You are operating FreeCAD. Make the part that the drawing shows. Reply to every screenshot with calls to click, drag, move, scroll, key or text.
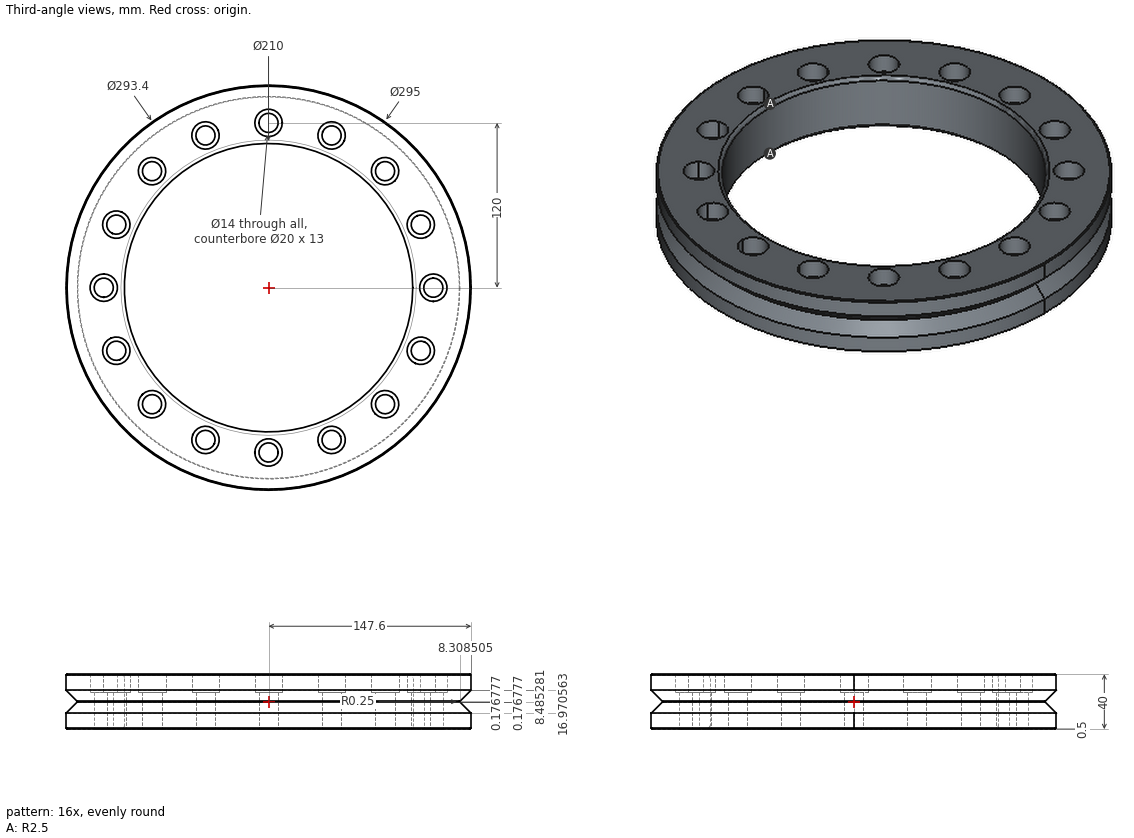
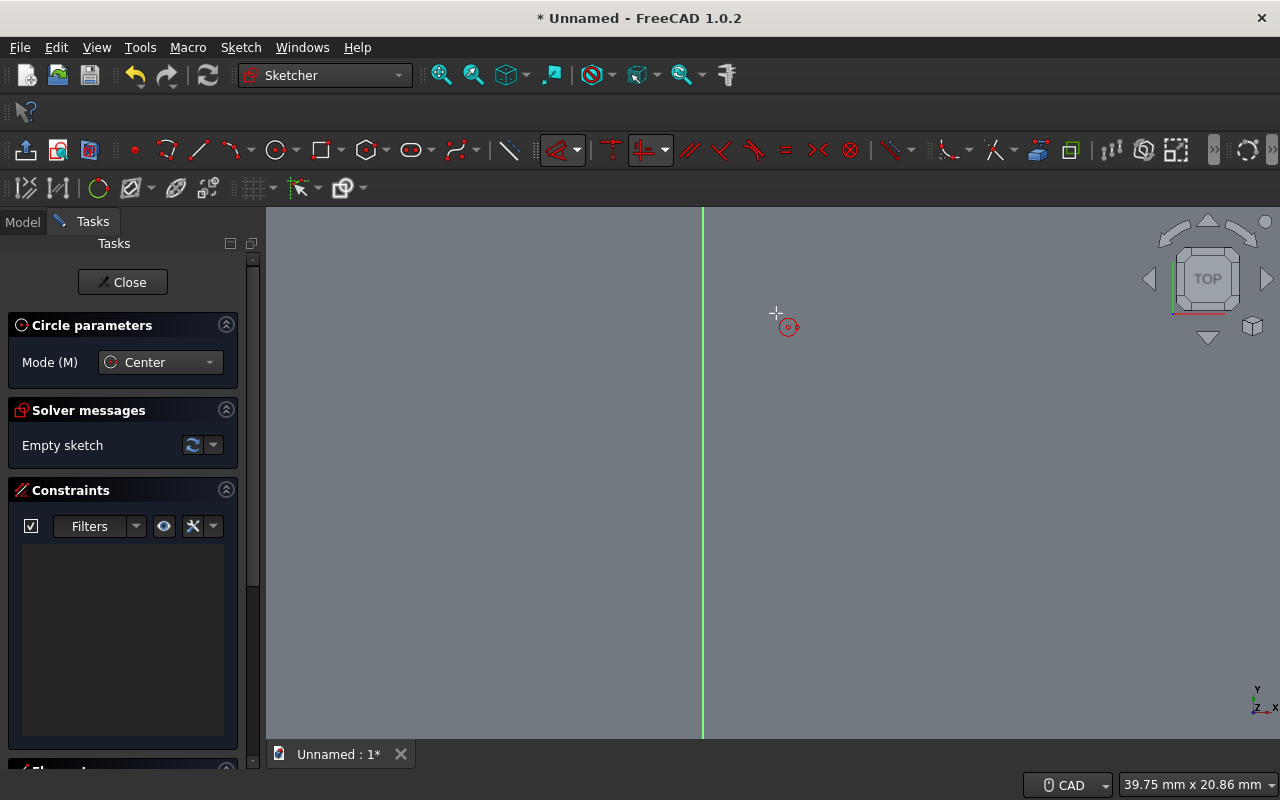
click(703, 462)
move(830, 335)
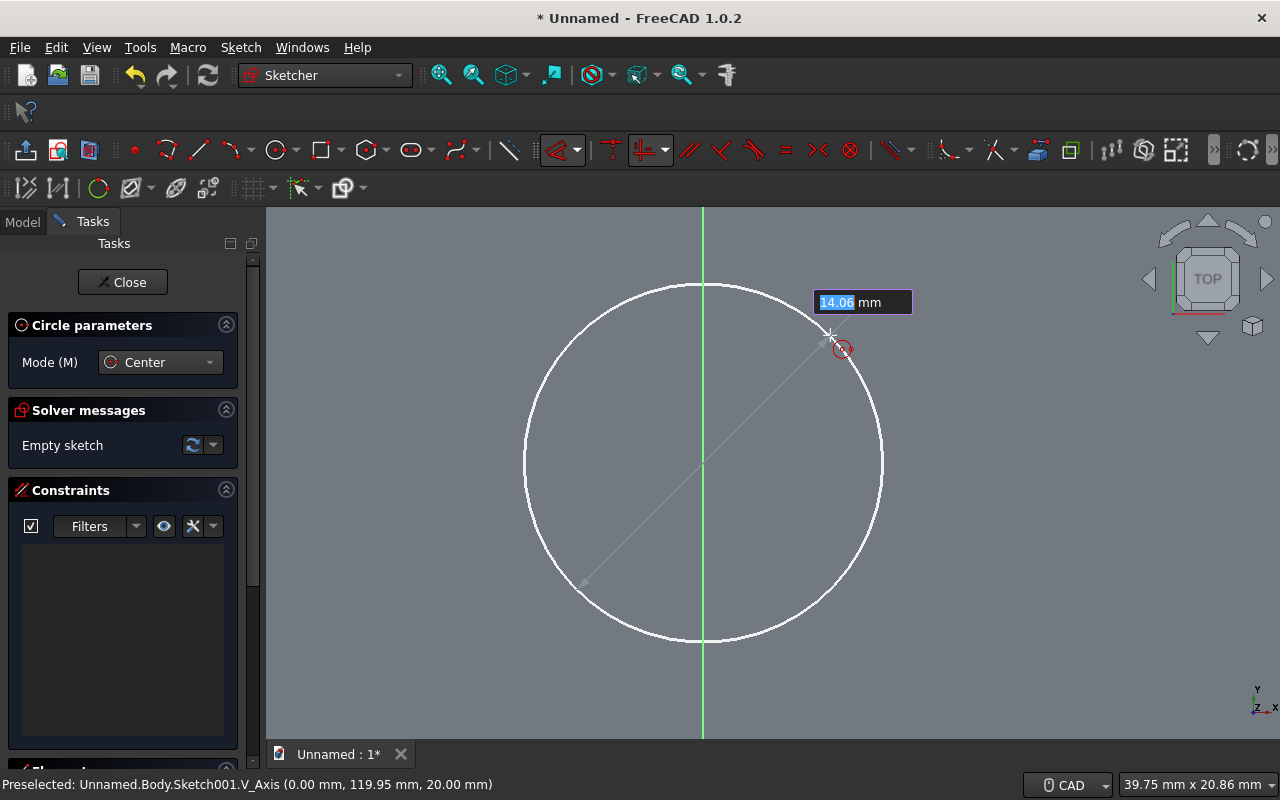
text(14)
key(Return)
key(Escape)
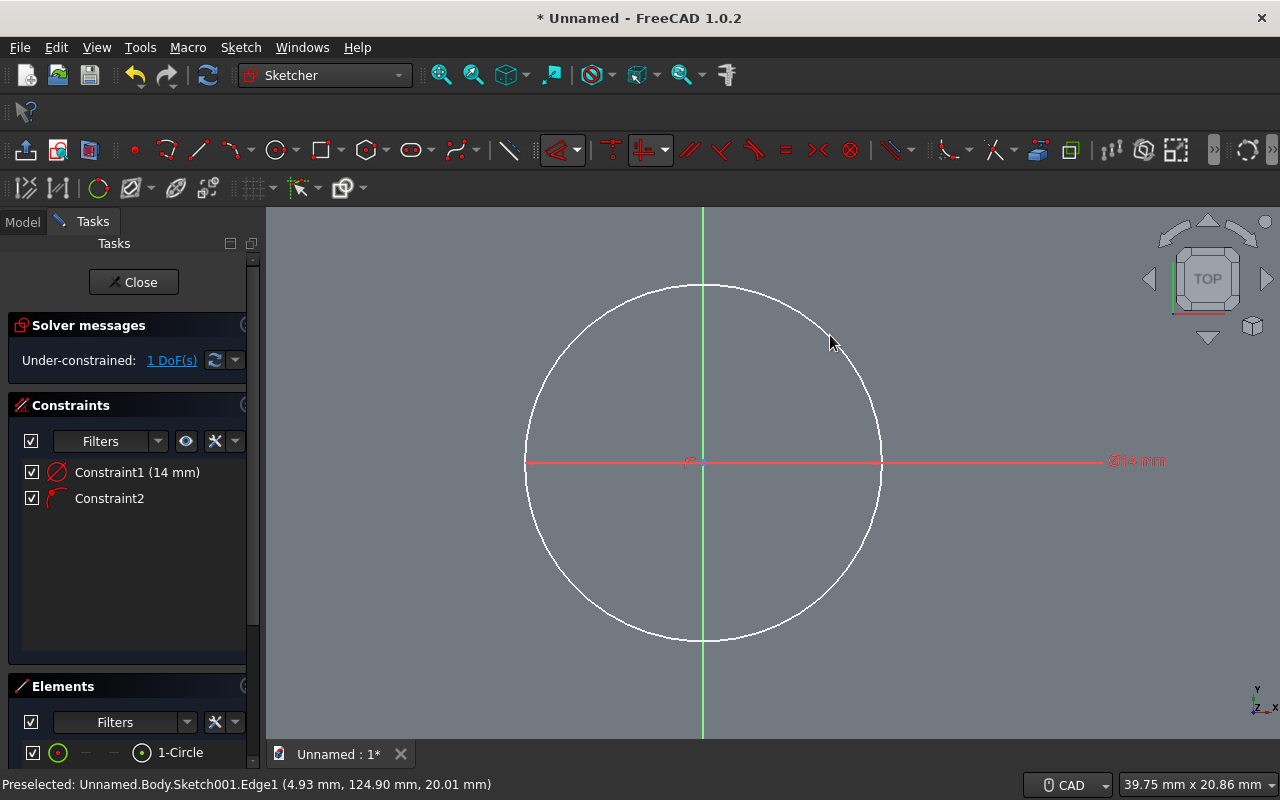
key(d)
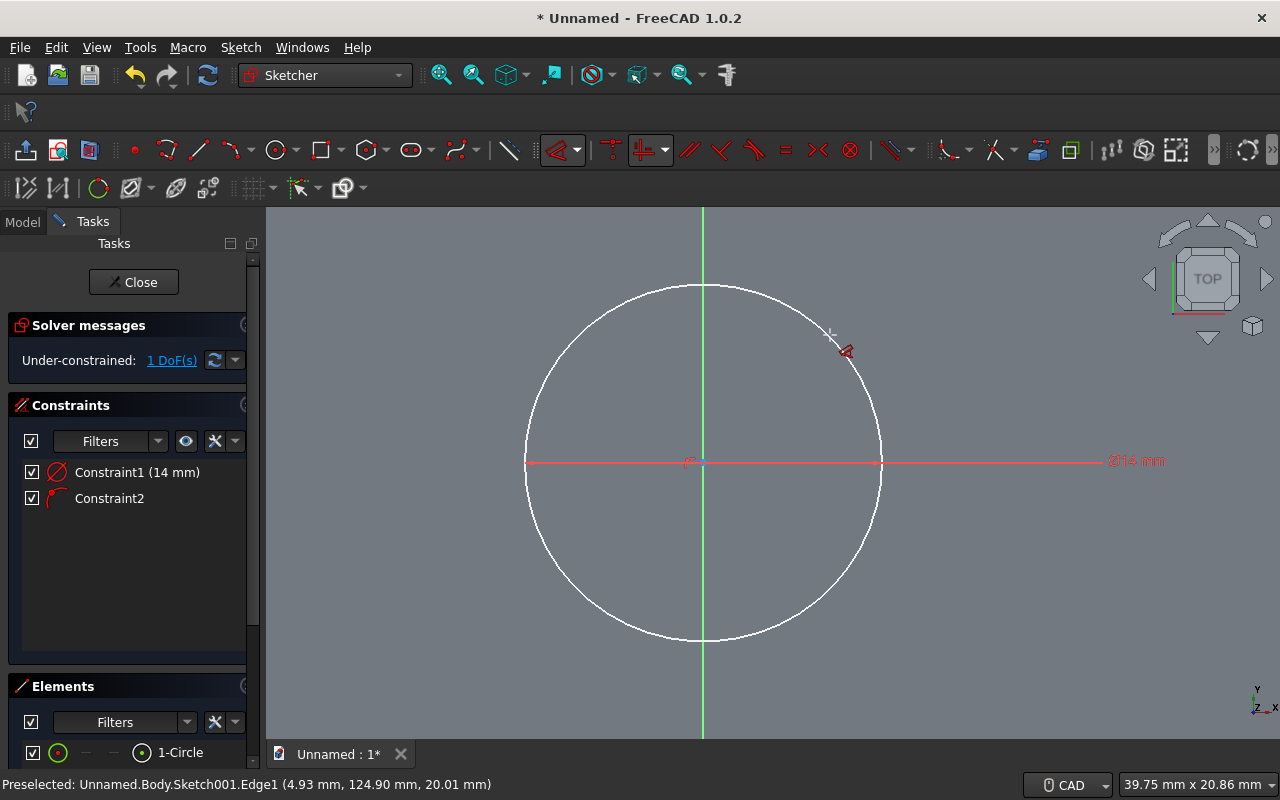
click(703, 463)
click(737, 587)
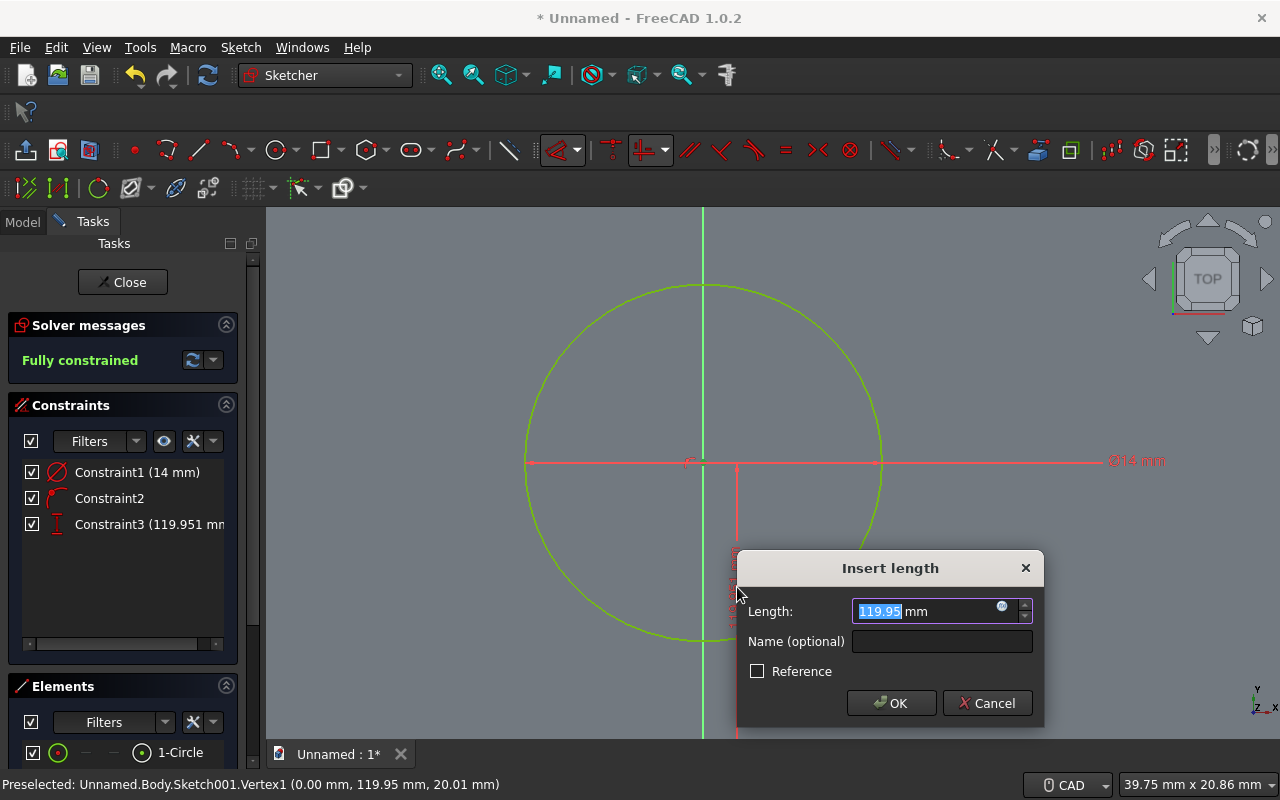
text(120)
key(Return)
key(Escape)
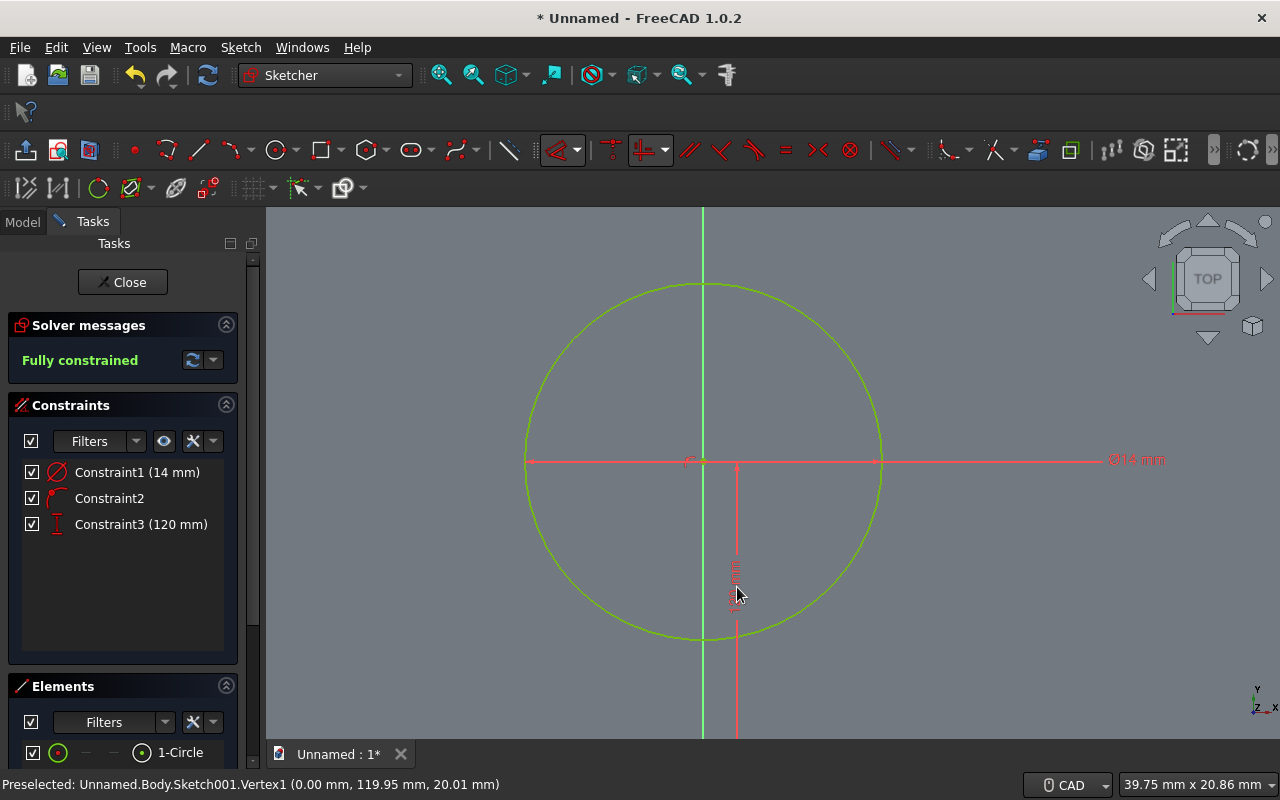
click(123, 282)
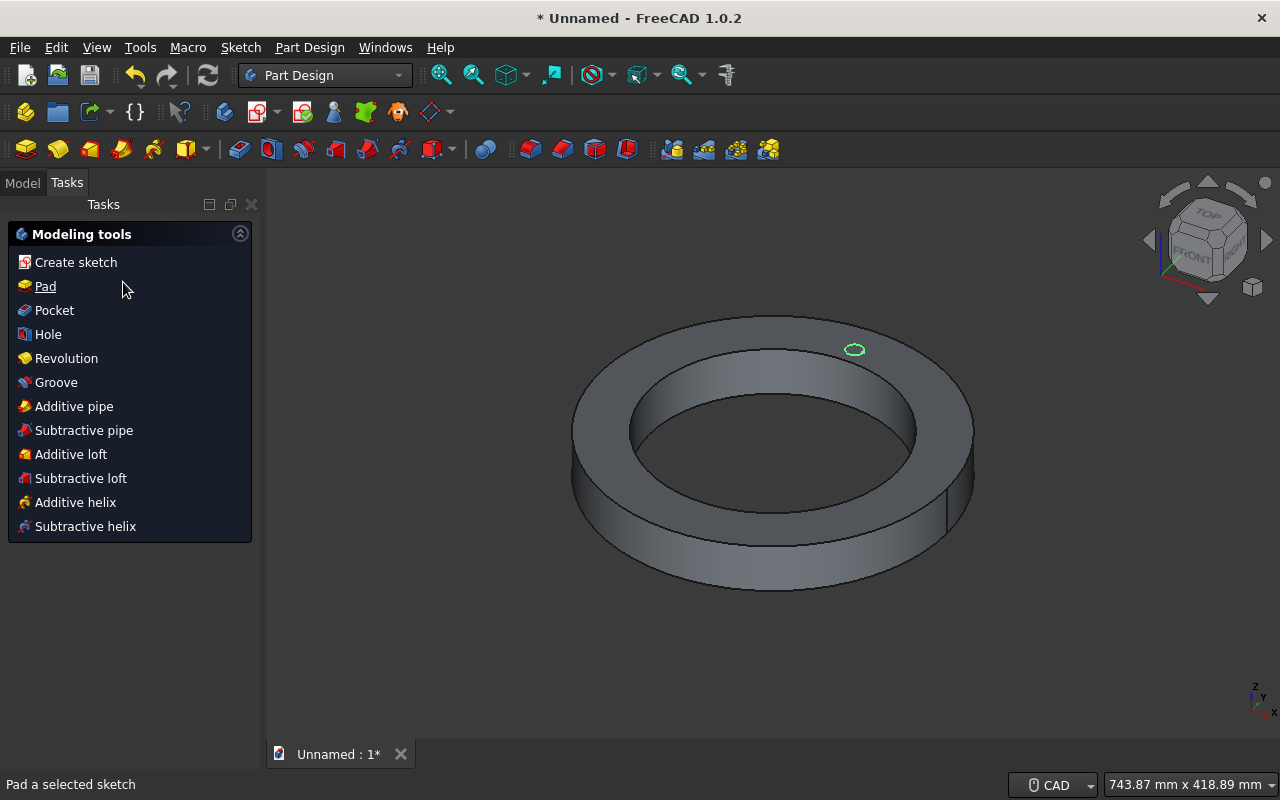
click(272, 150)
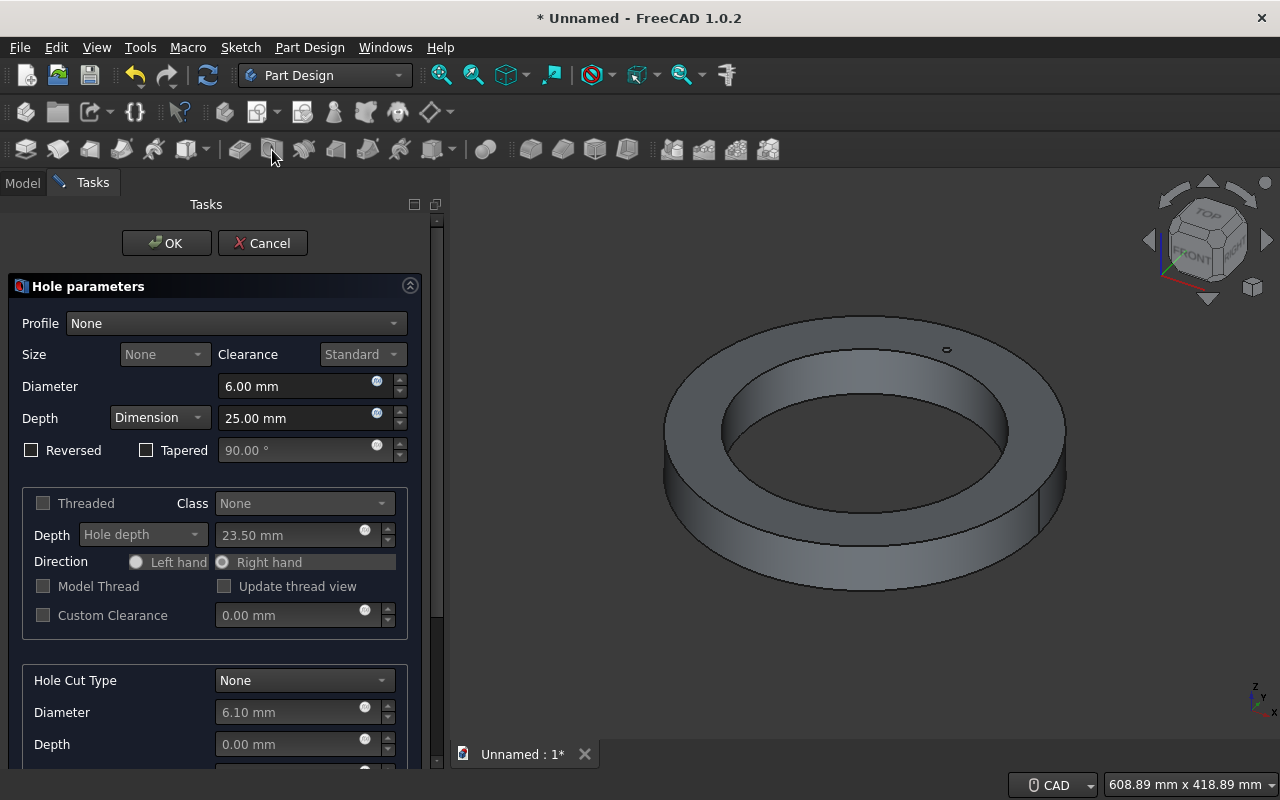
triple_click(305, 386)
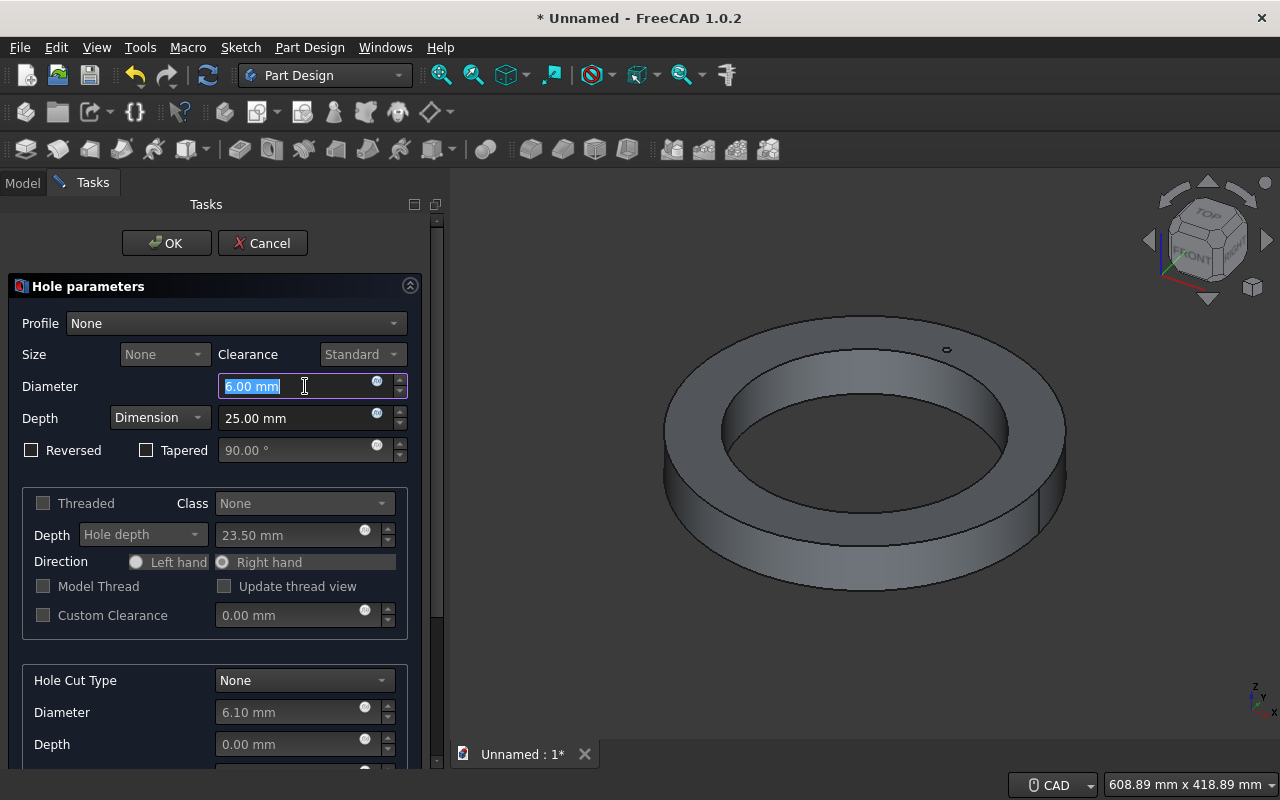
text(14)
key(Tab)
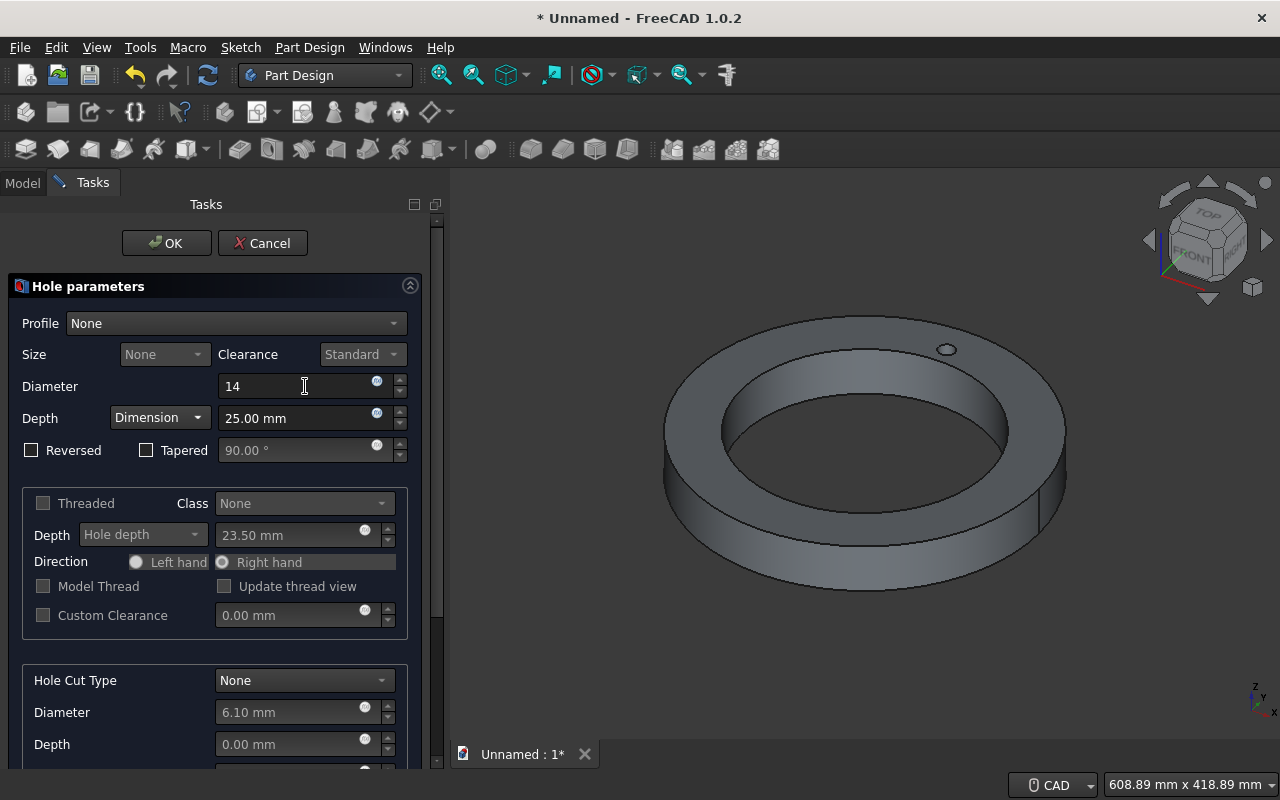
click(161, 418)